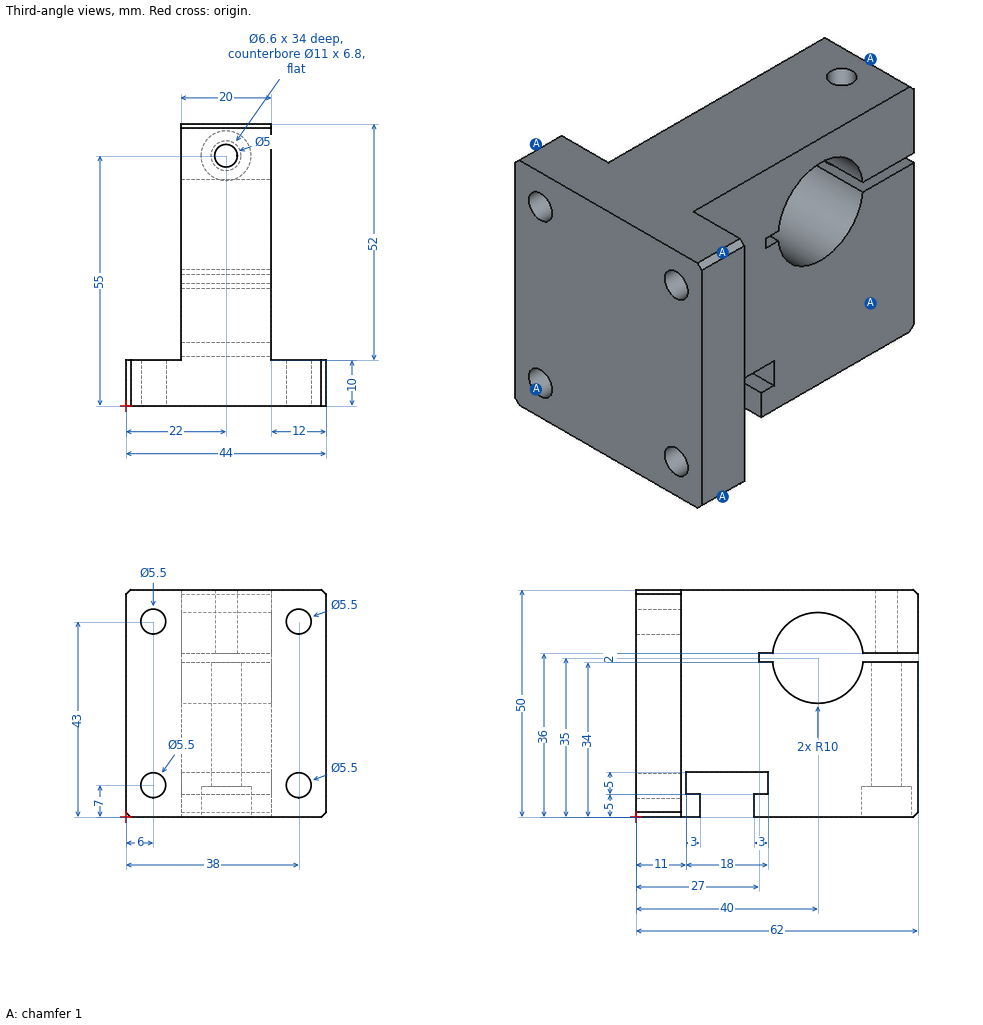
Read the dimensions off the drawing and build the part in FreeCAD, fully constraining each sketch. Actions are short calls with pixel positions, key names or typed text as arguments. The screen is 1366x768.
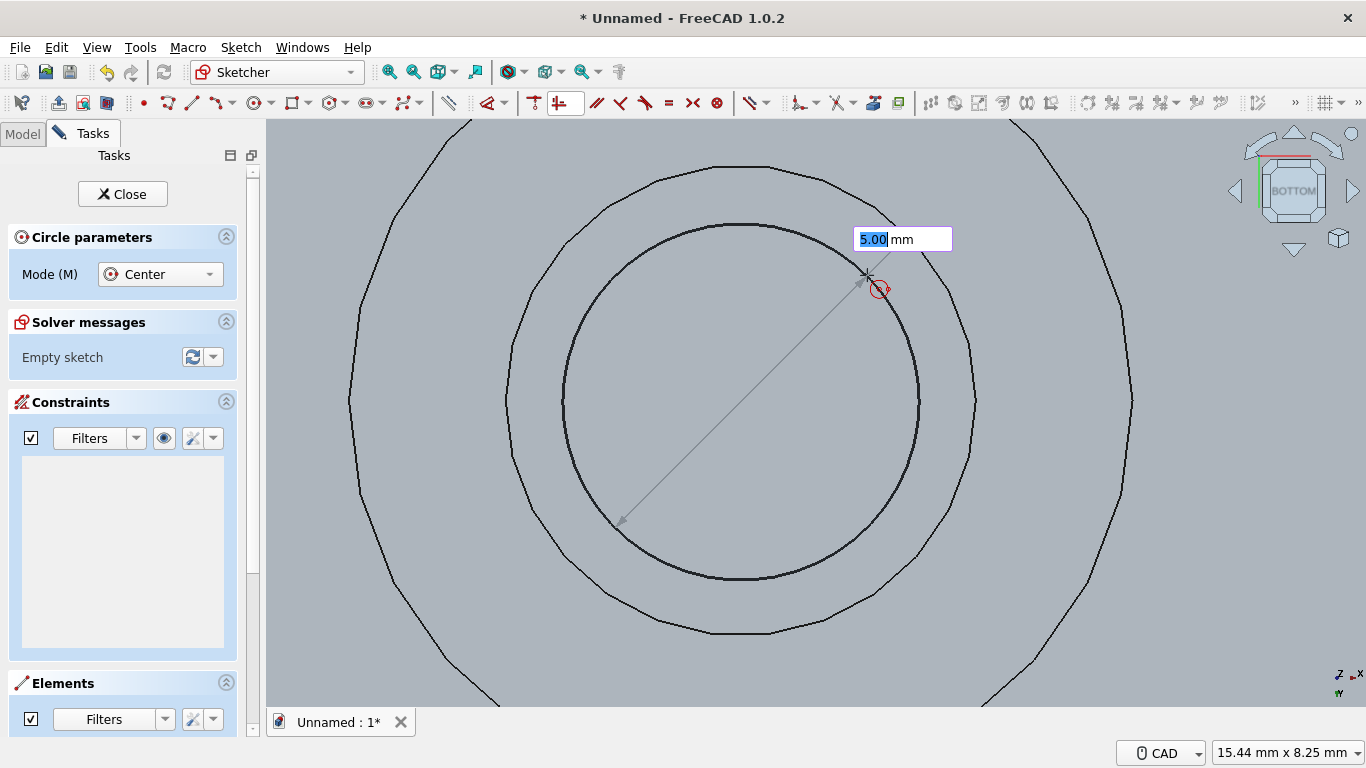
text(5)
key(Return)
key(Escape)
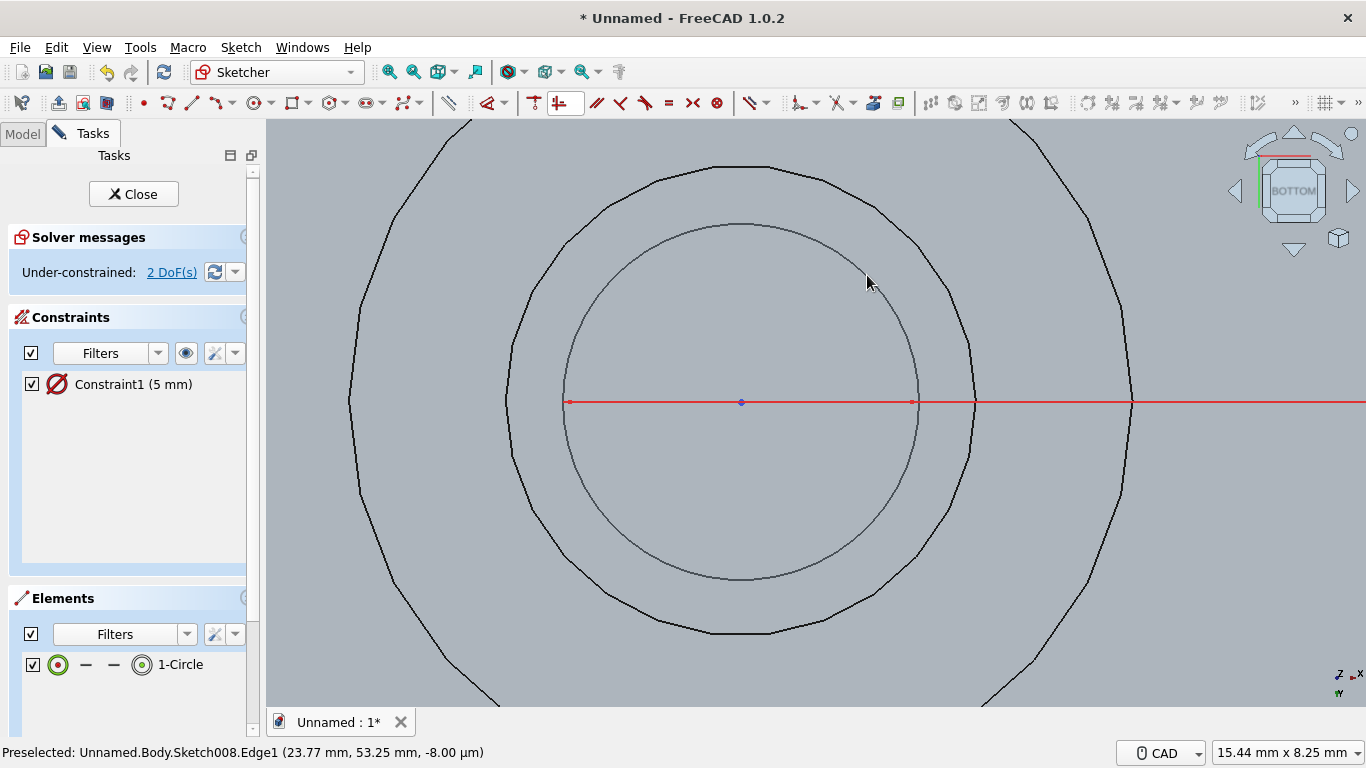
click(488, 104)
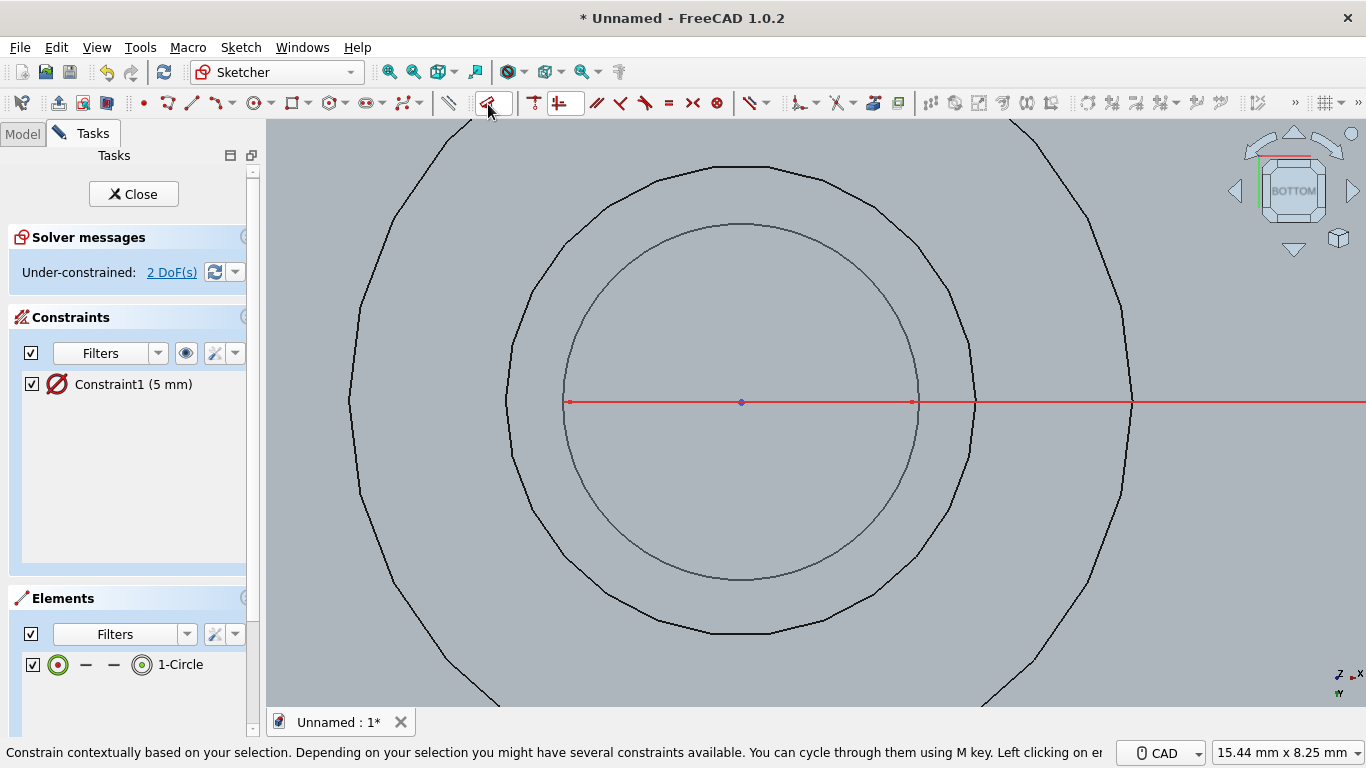
click(741, 402)
click(517, 436)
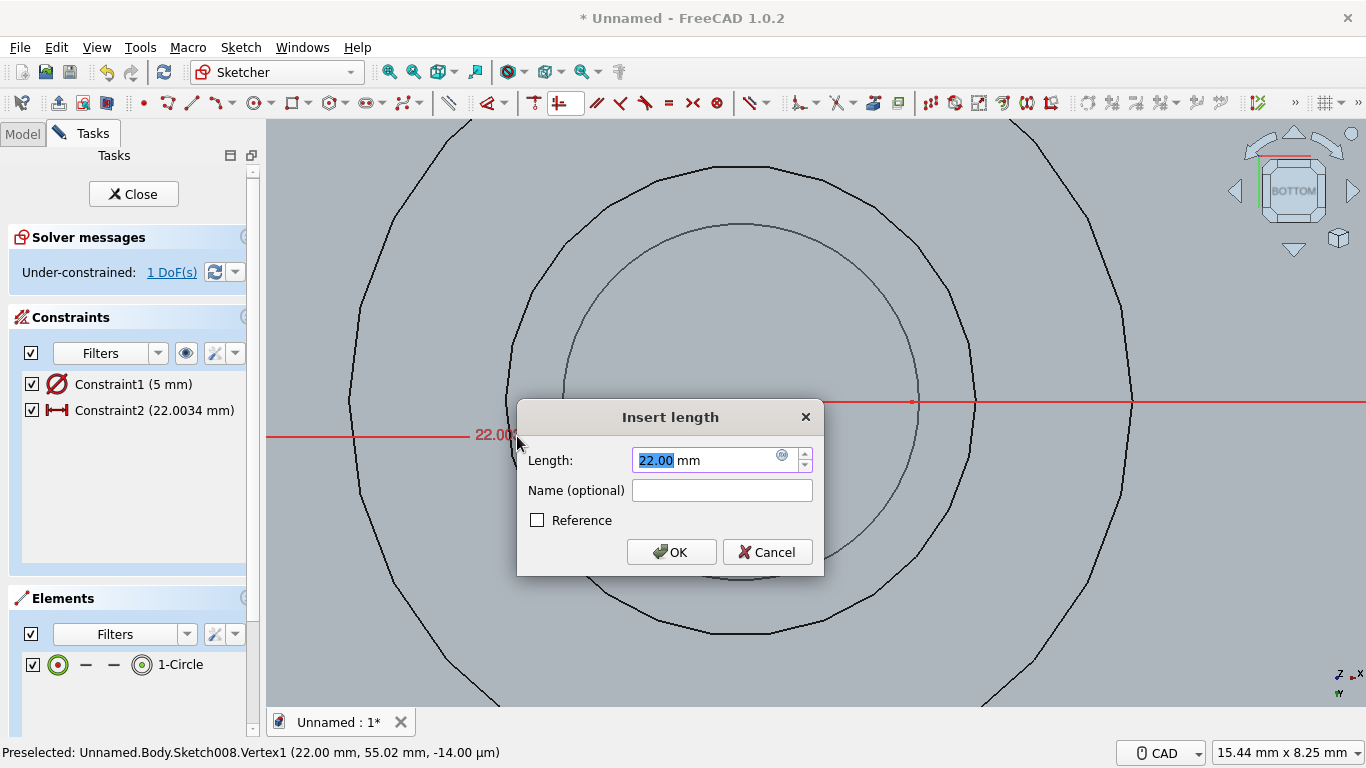
text(22)
key(Return)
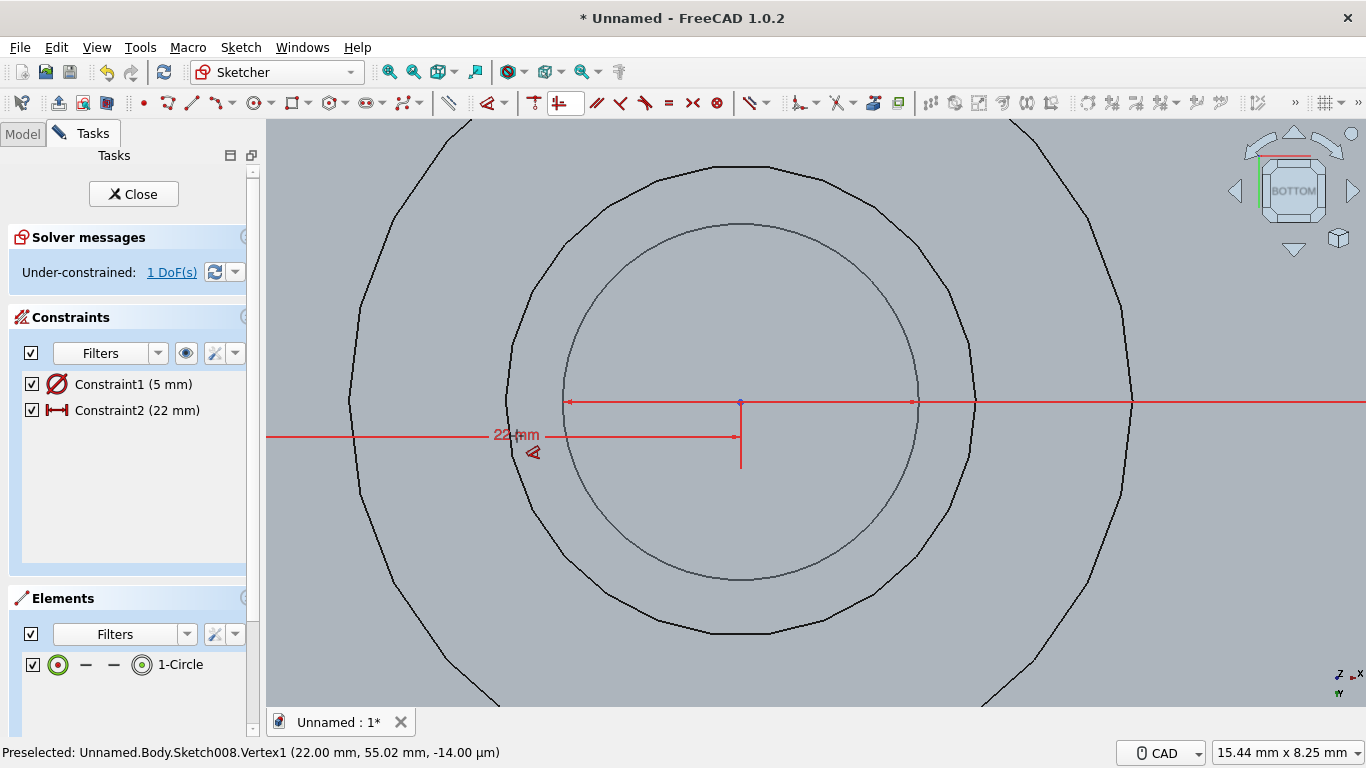
click(741, 402)
click(775, 275)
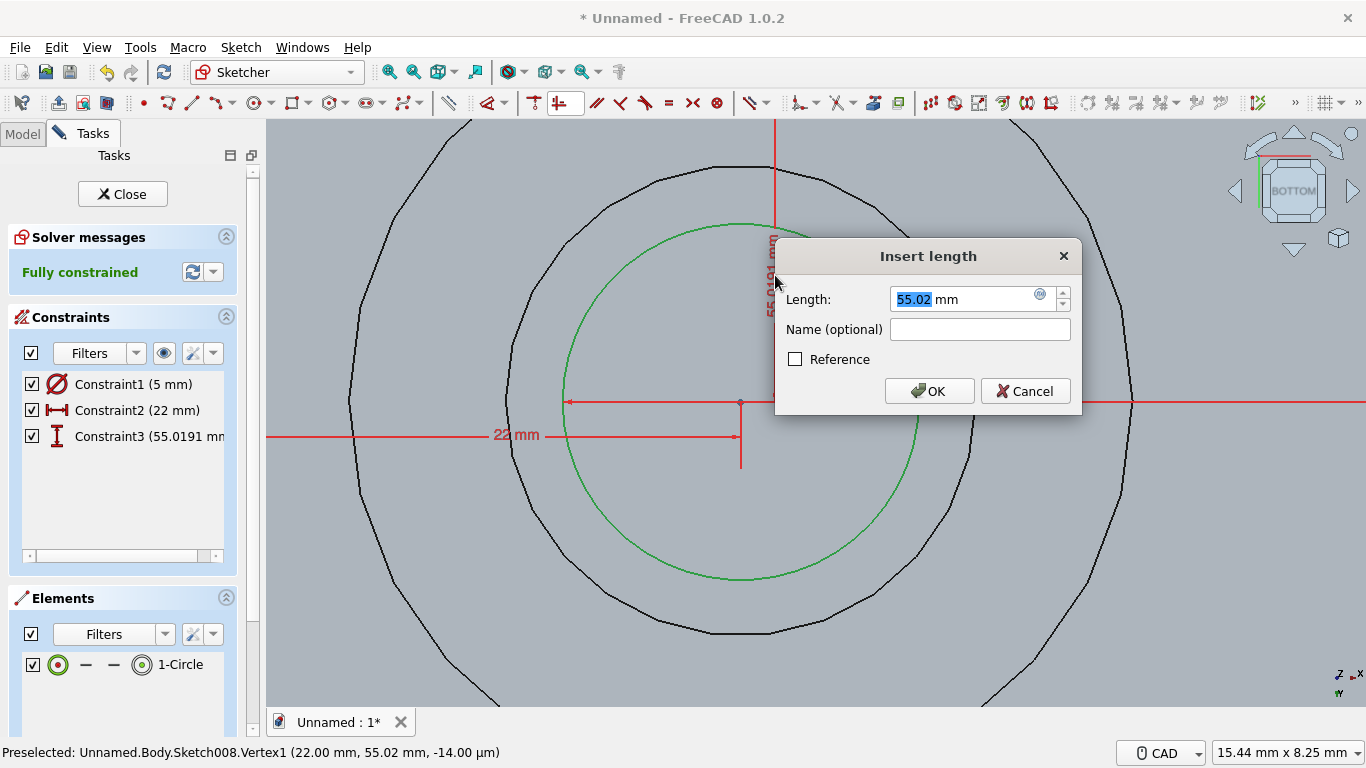
text(55)
key(Return)
key(Escape)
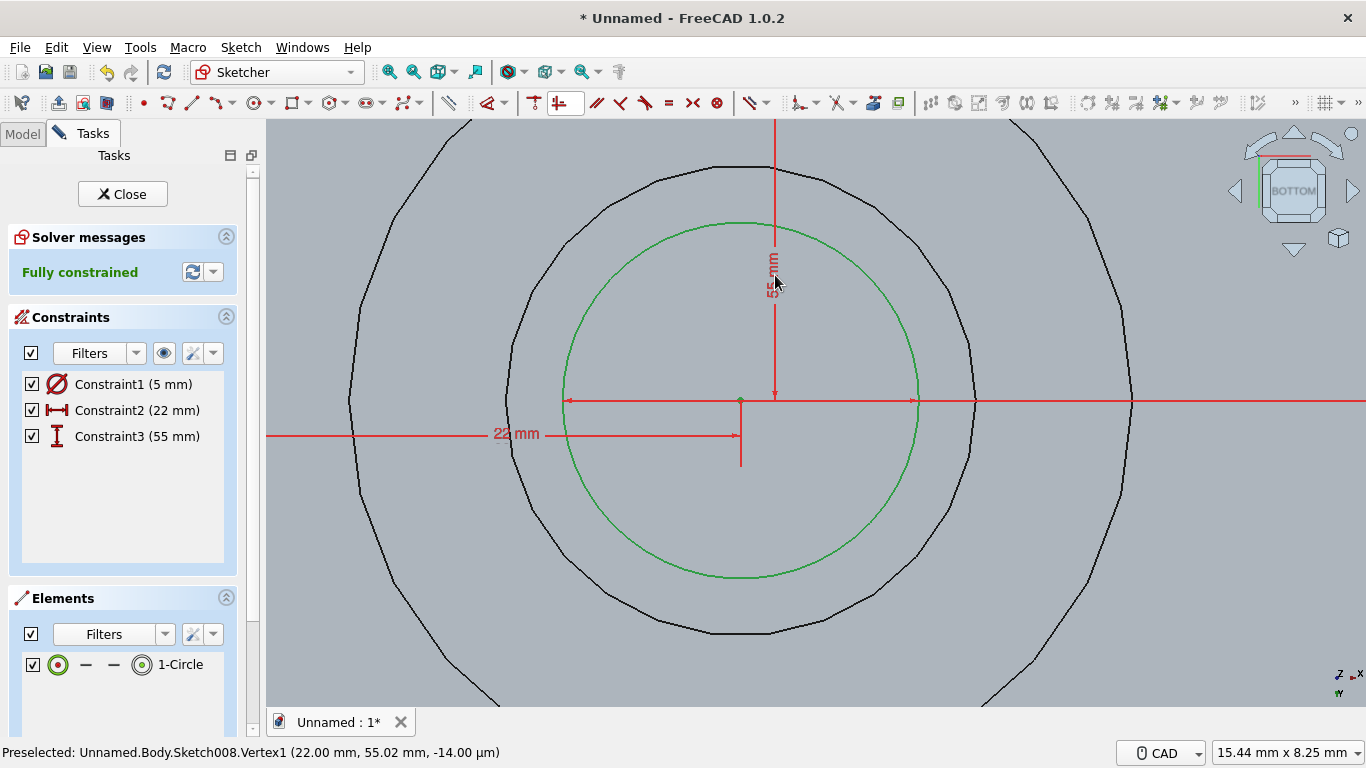
click(123, 194)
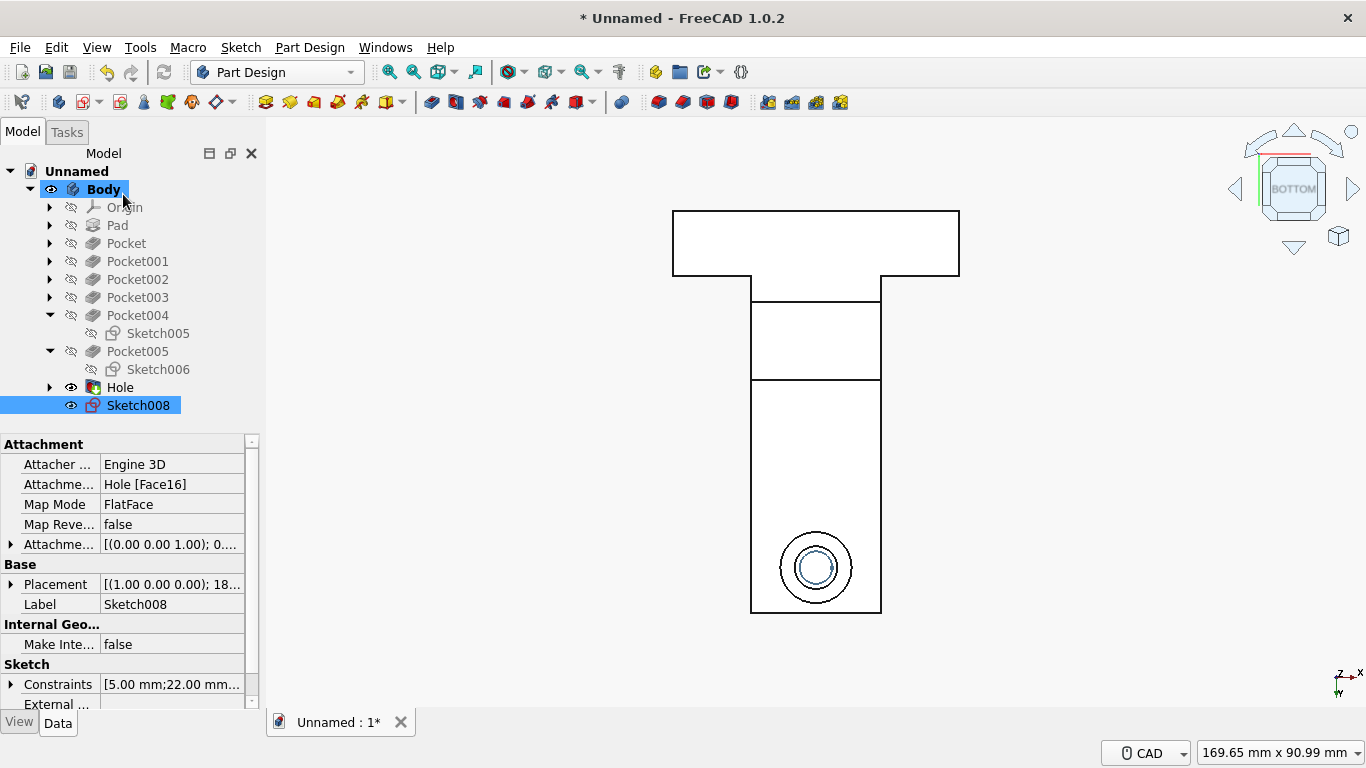
click(432, 102)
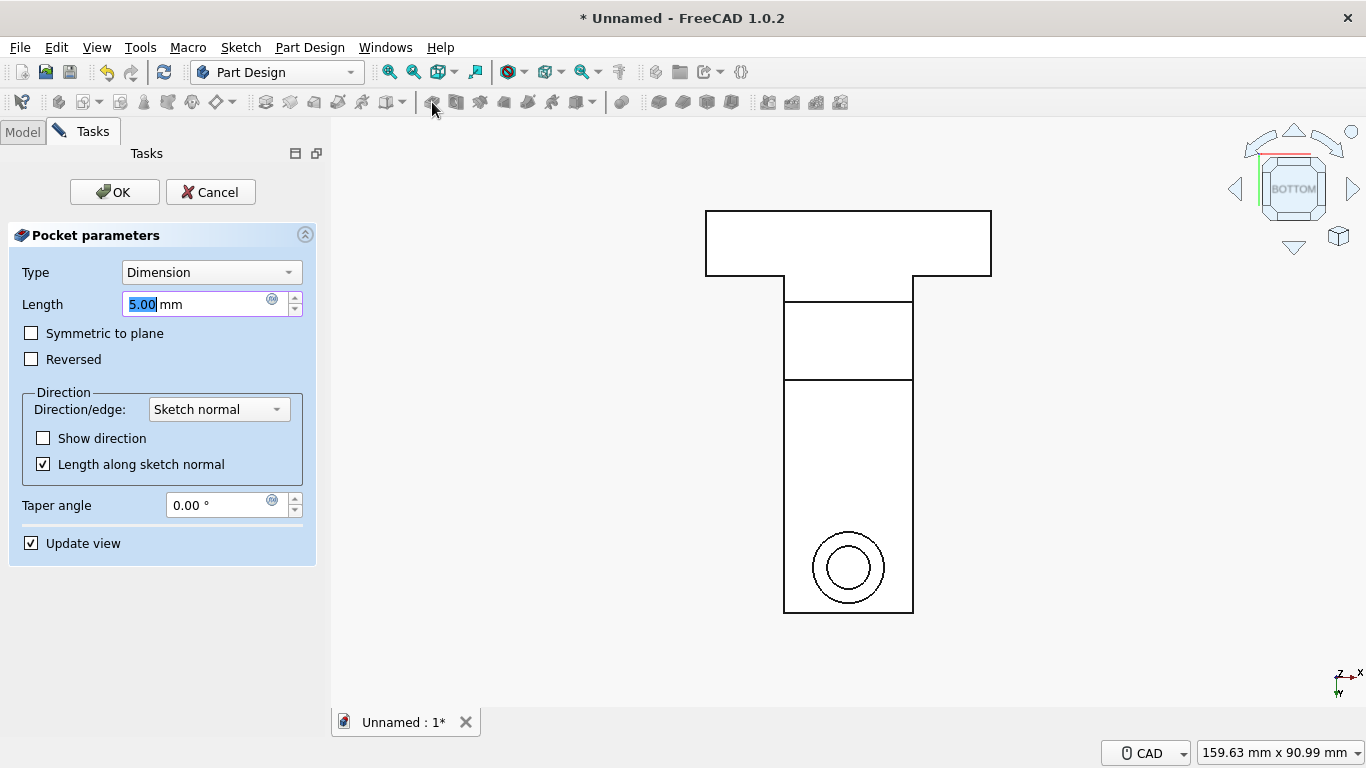
click(212, 272)